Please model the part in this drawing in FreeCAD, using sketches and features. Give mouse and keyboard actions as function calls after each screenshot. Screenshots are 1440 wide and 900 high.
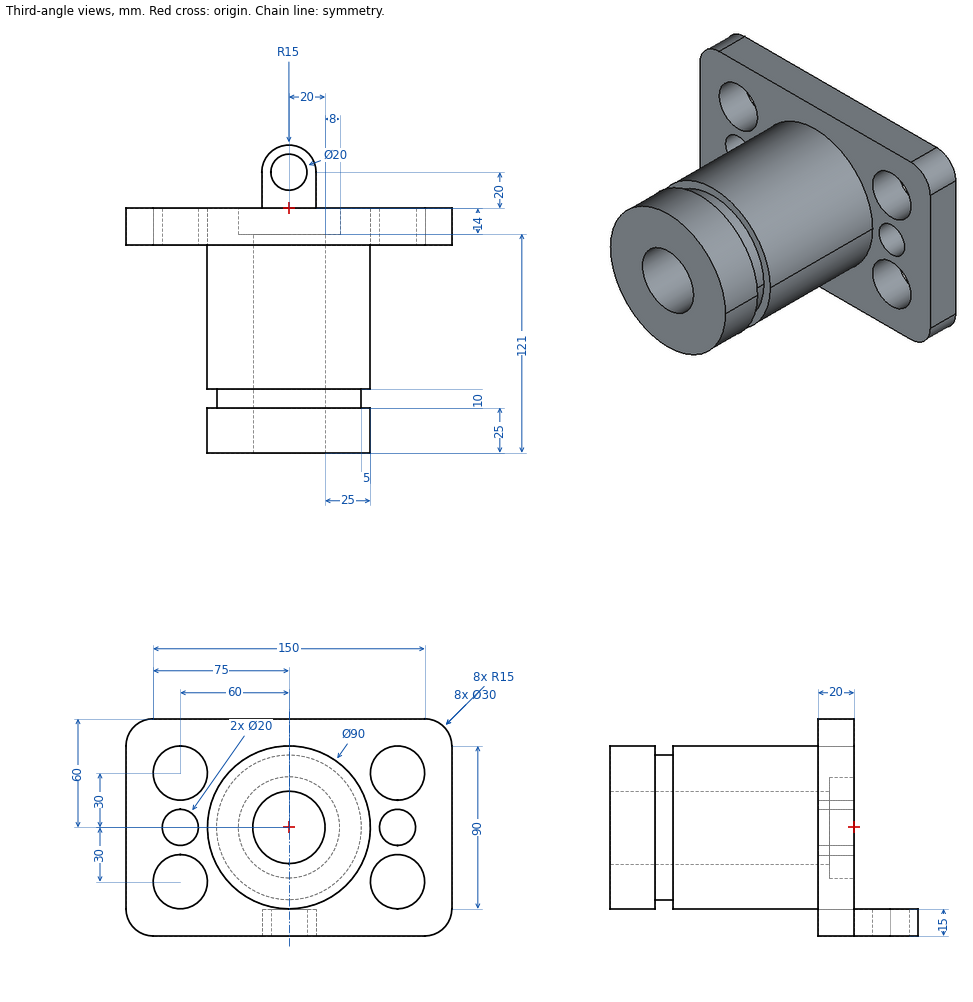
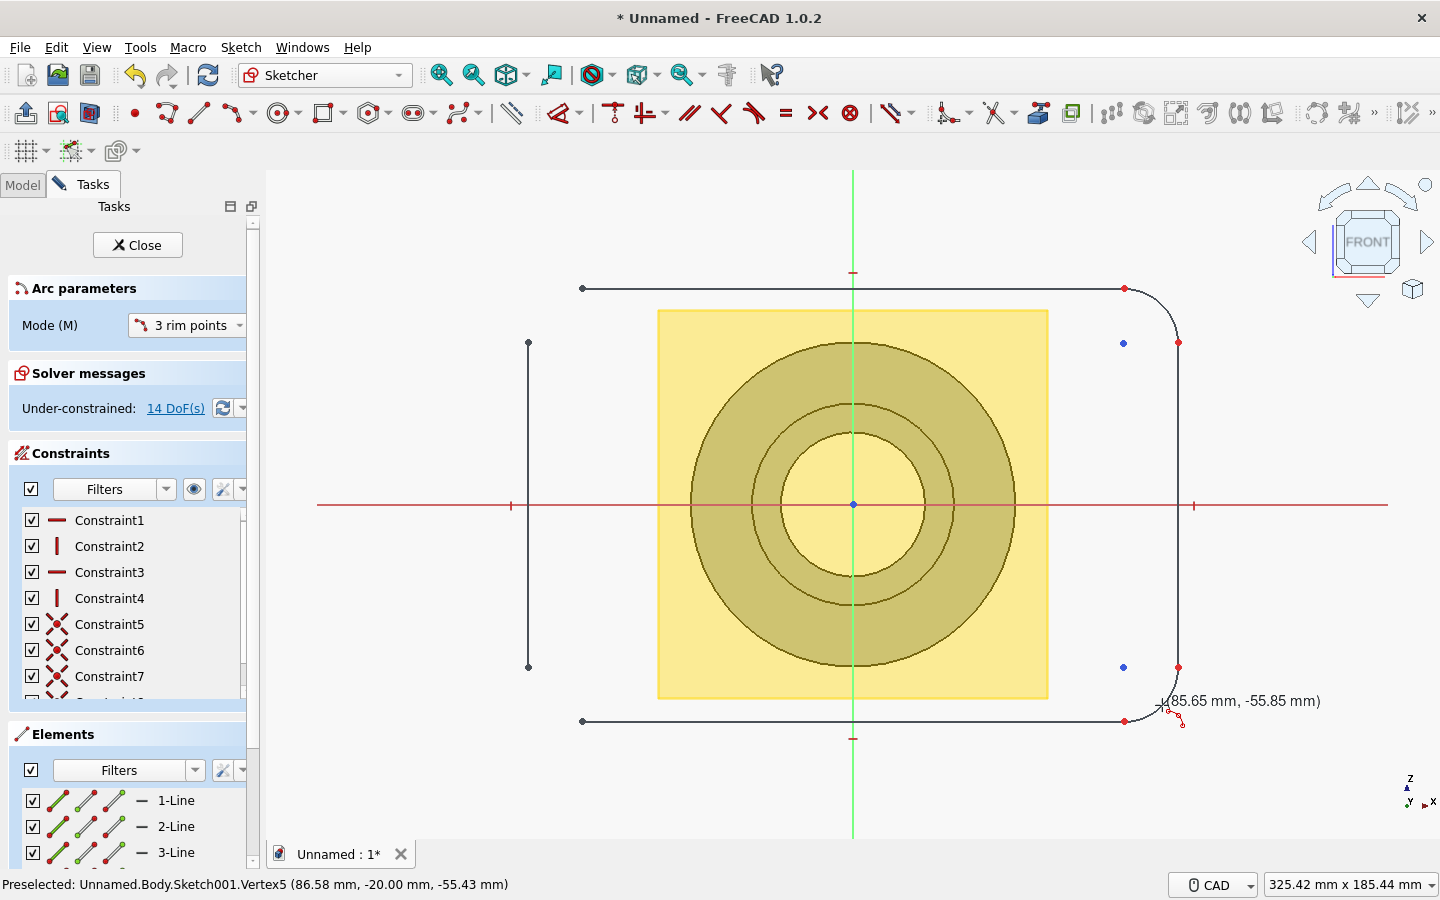
click(582, 722)
click(528, 668)
click(544, 705)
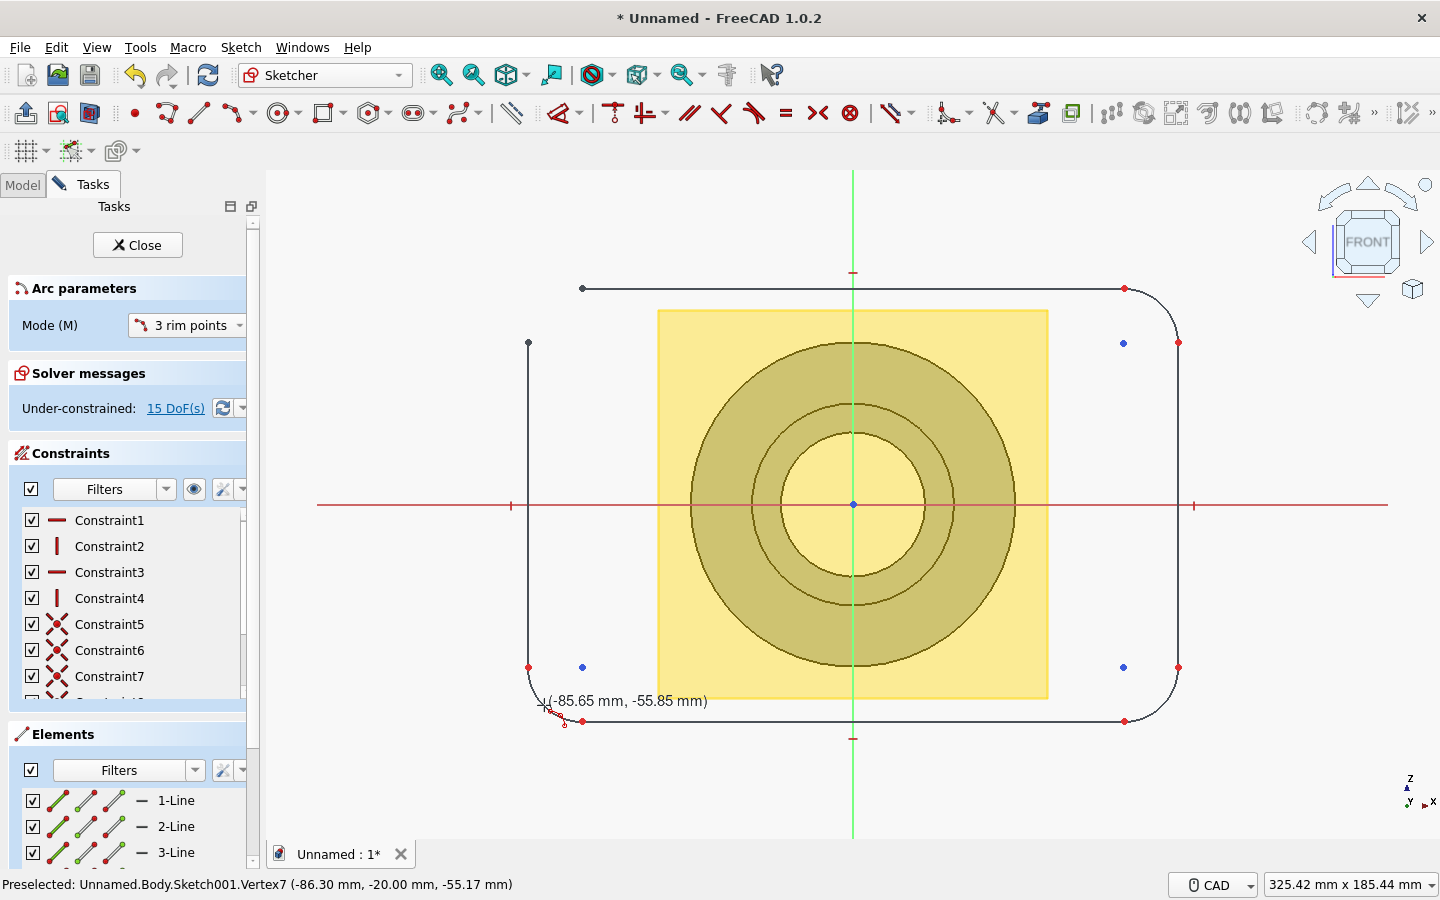
click(528, 343)
click(582, 289)
click(544, 304)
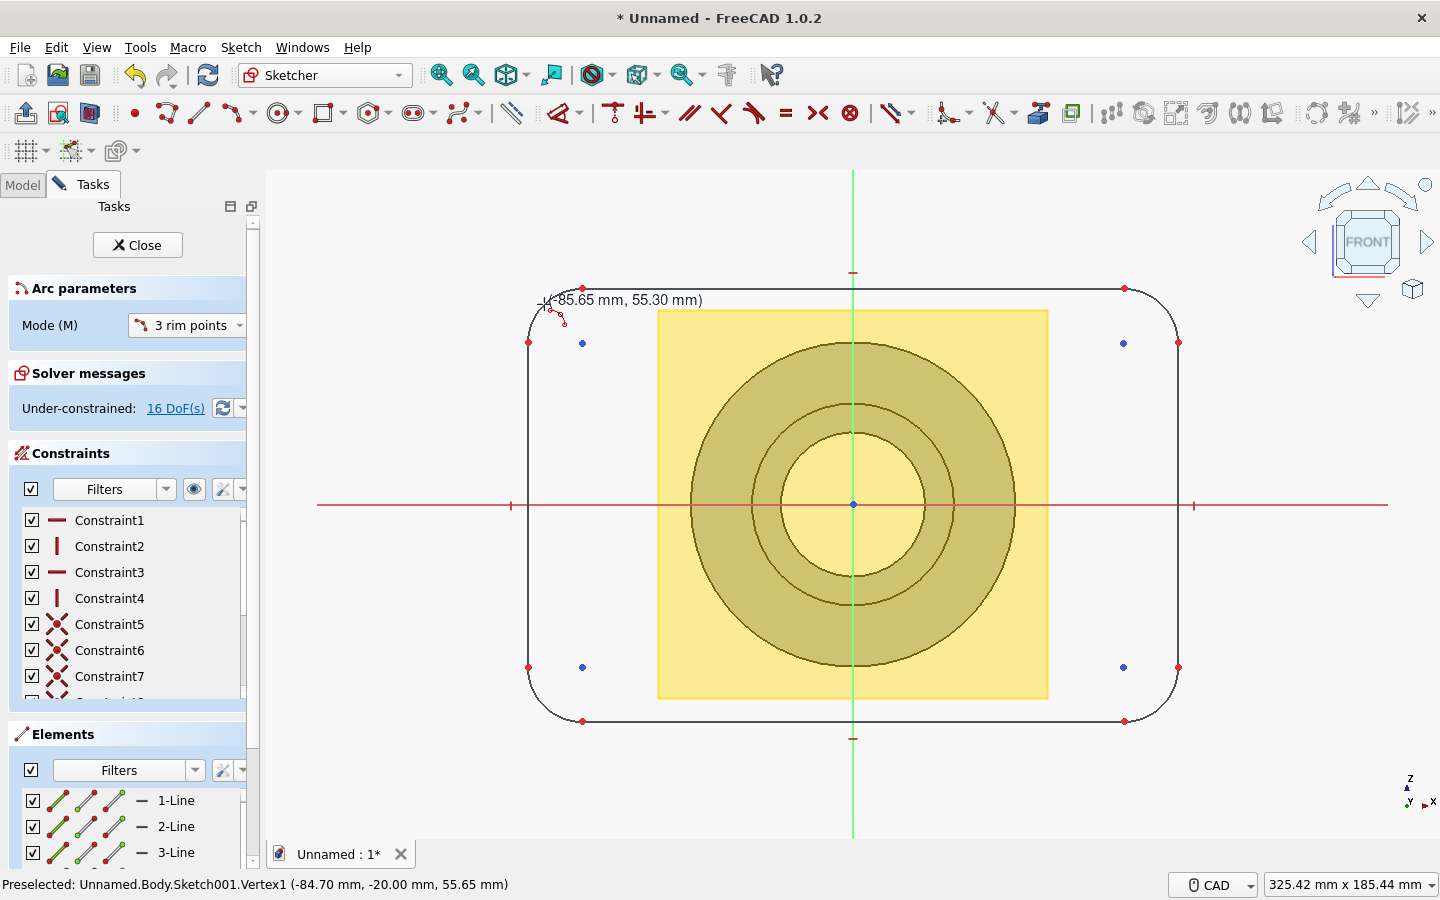
click(278, 114)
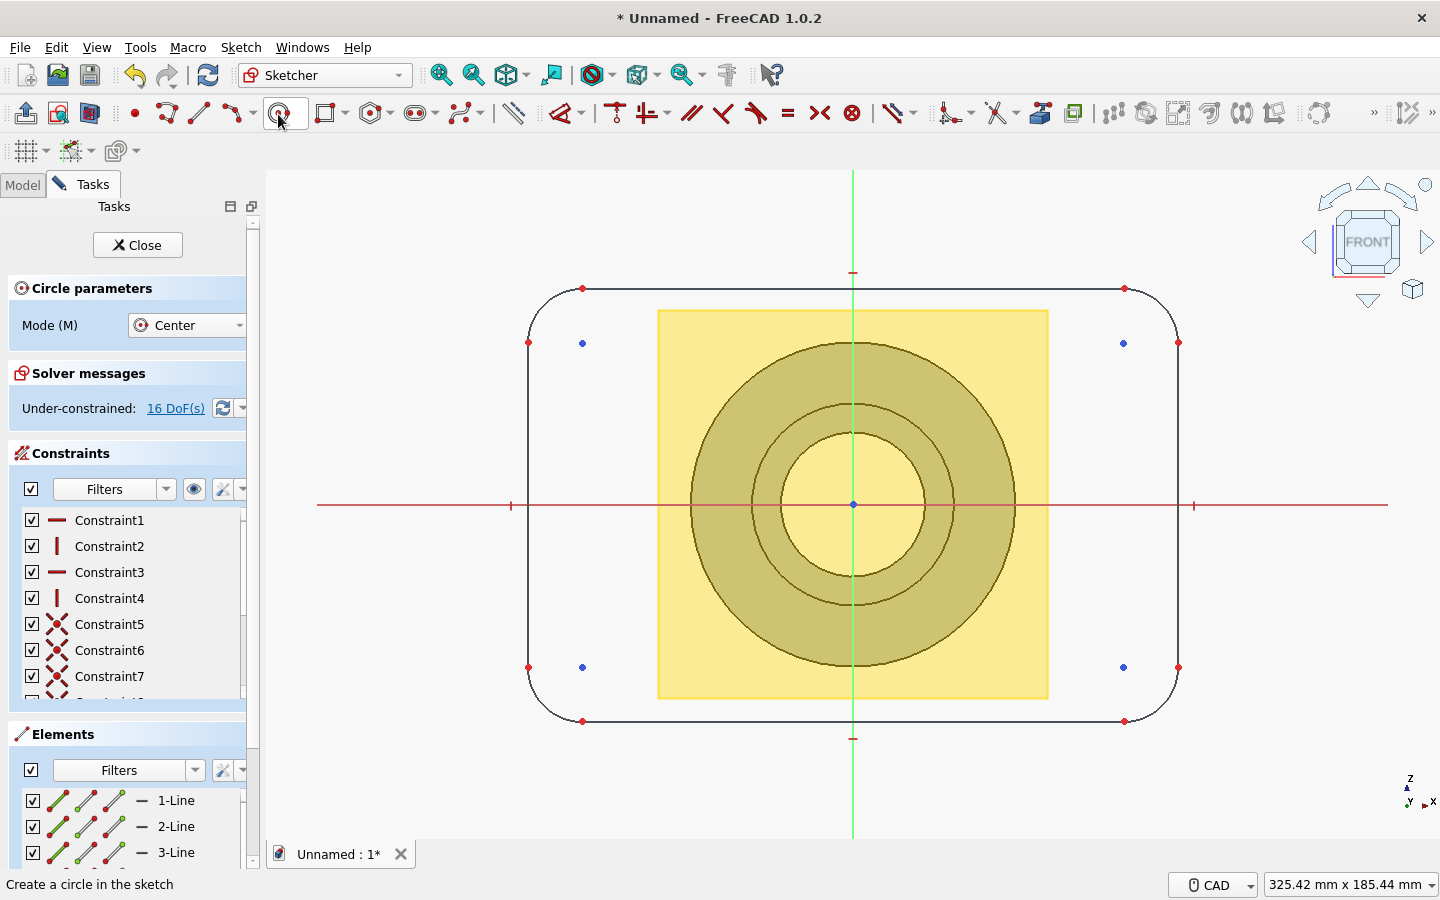
click(637, 396)
move(675, 358)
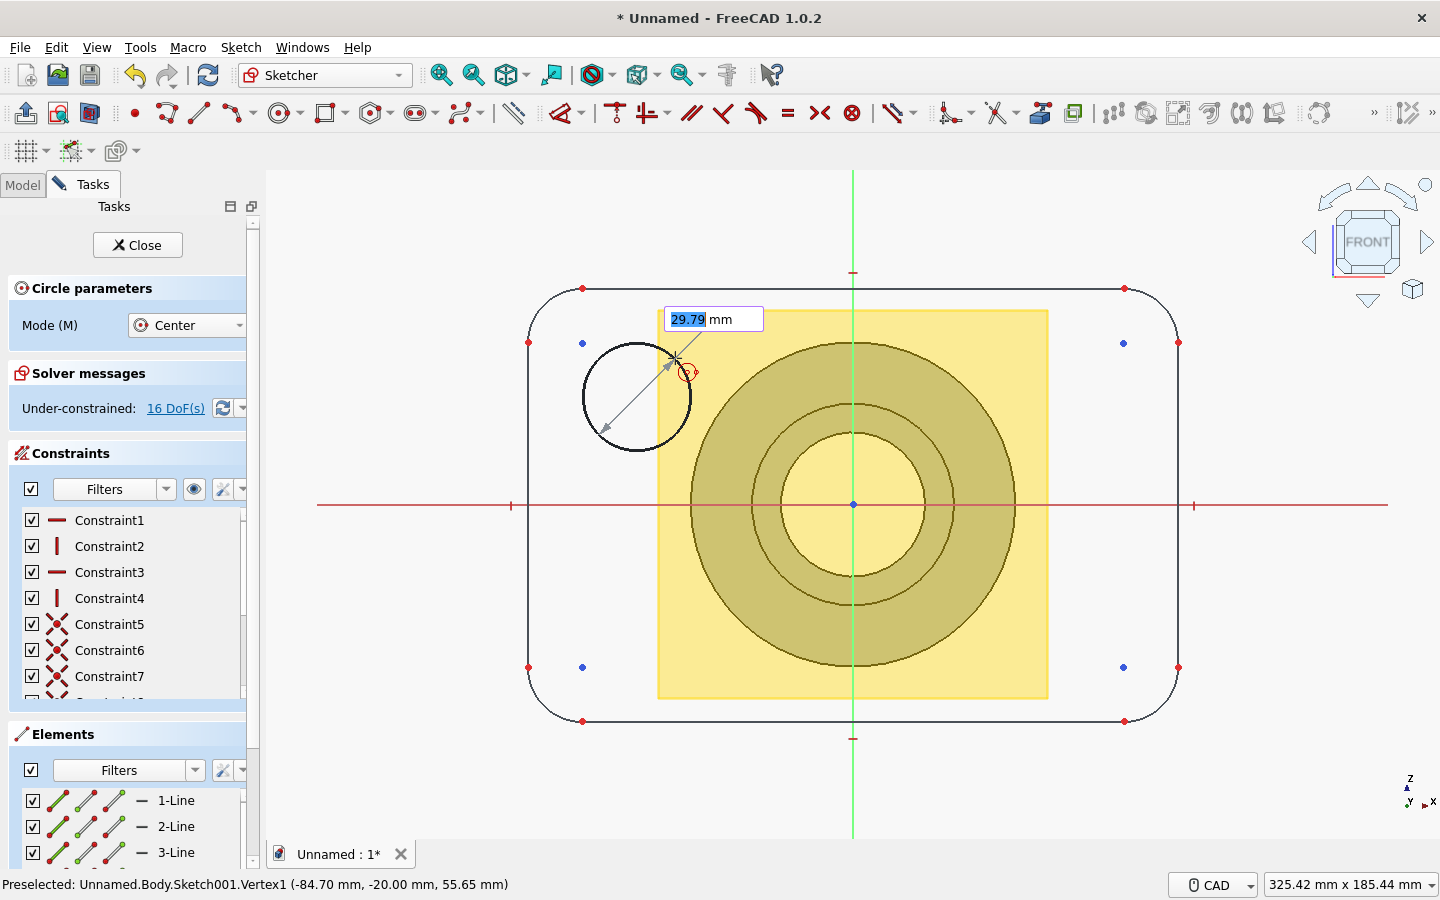
text(30)
key(Return)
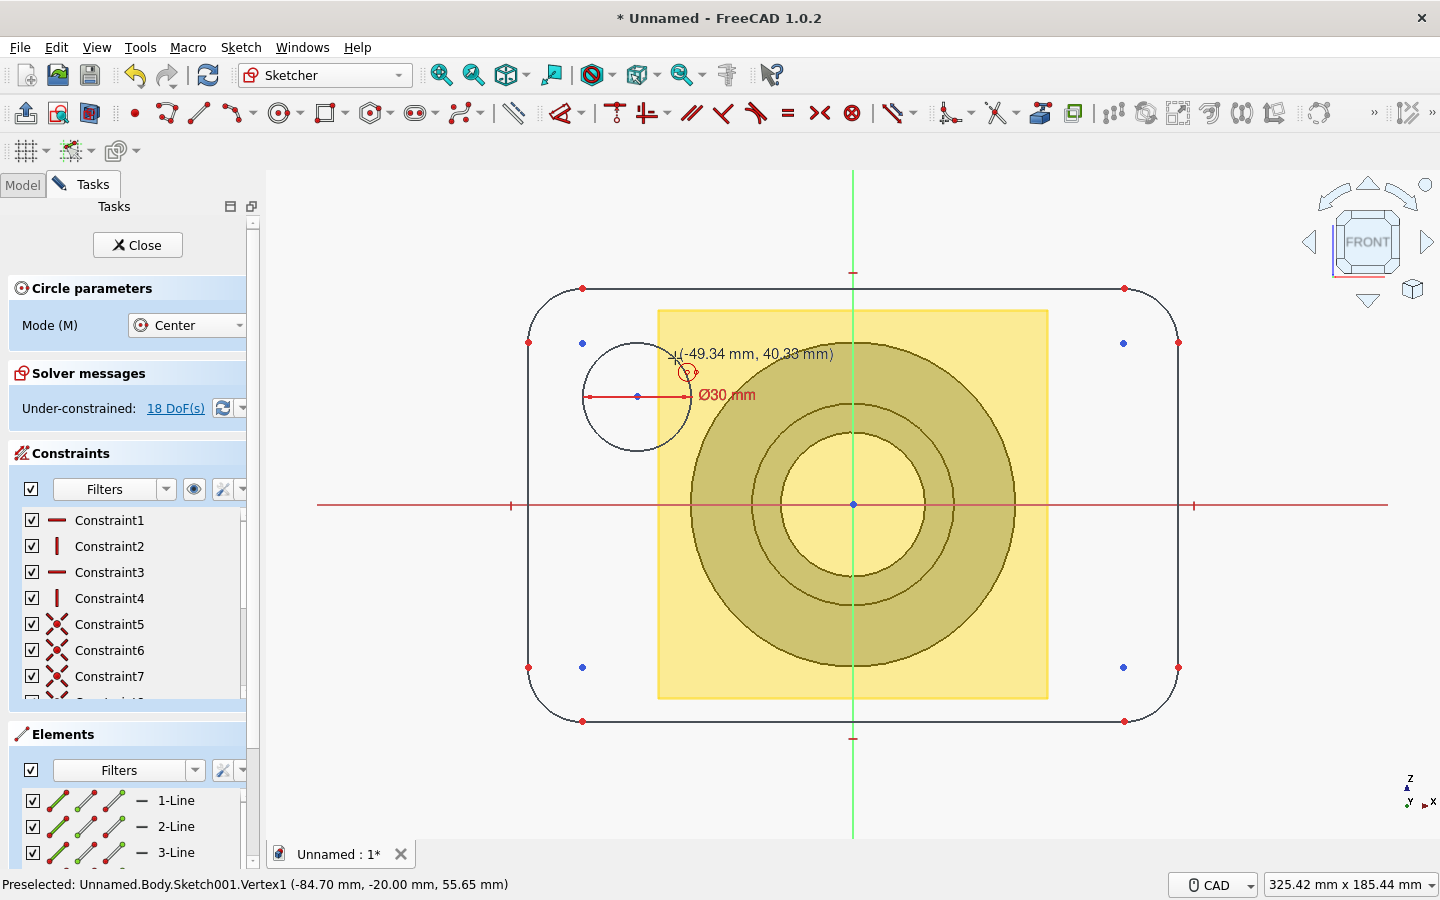
click(1069, 396)
move(1108, 358)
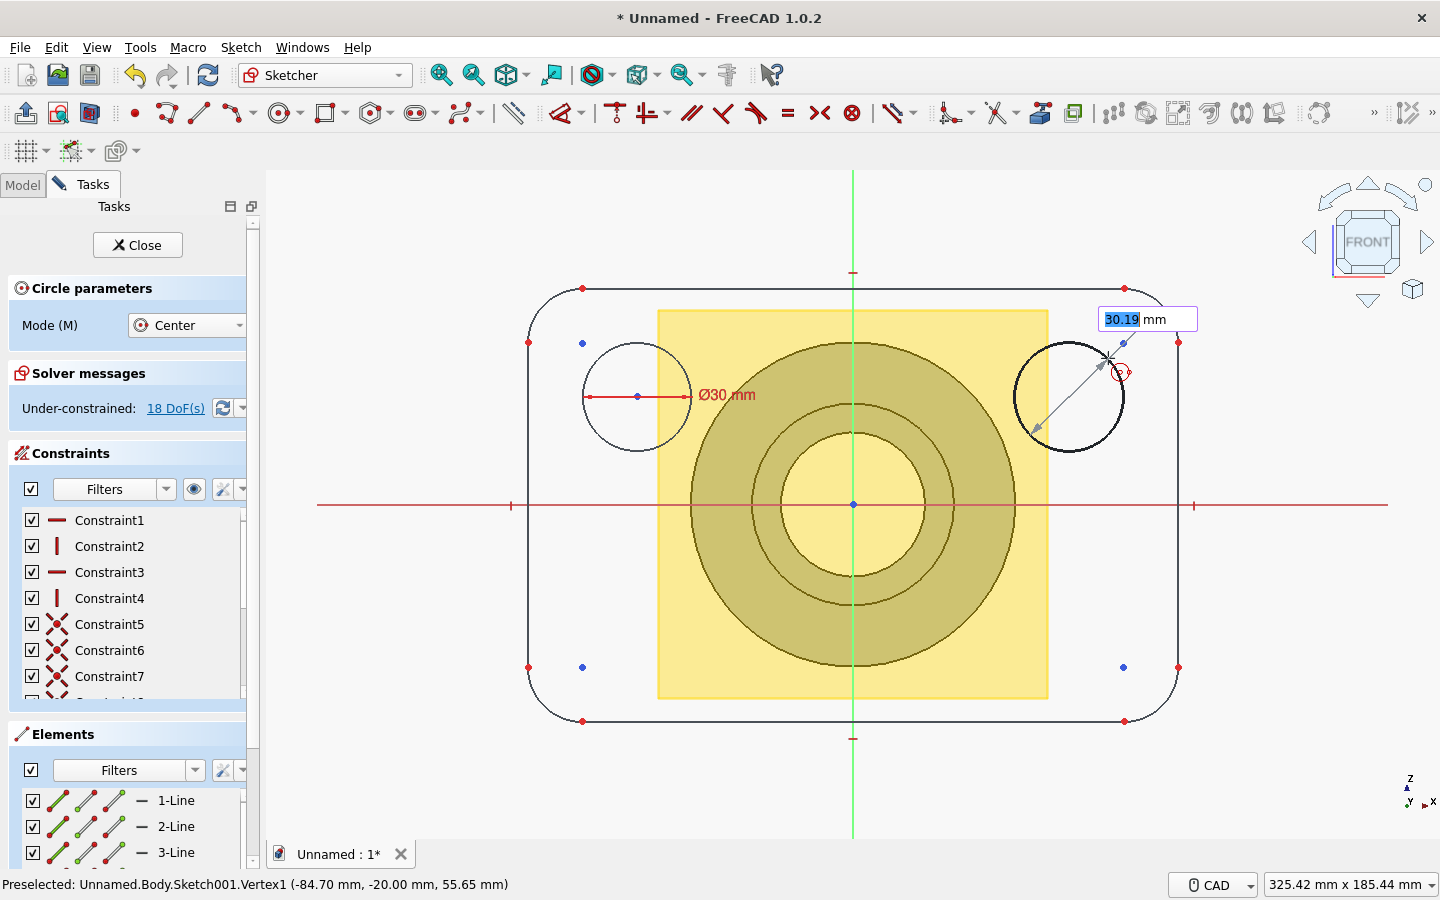
text(30)
key(Return)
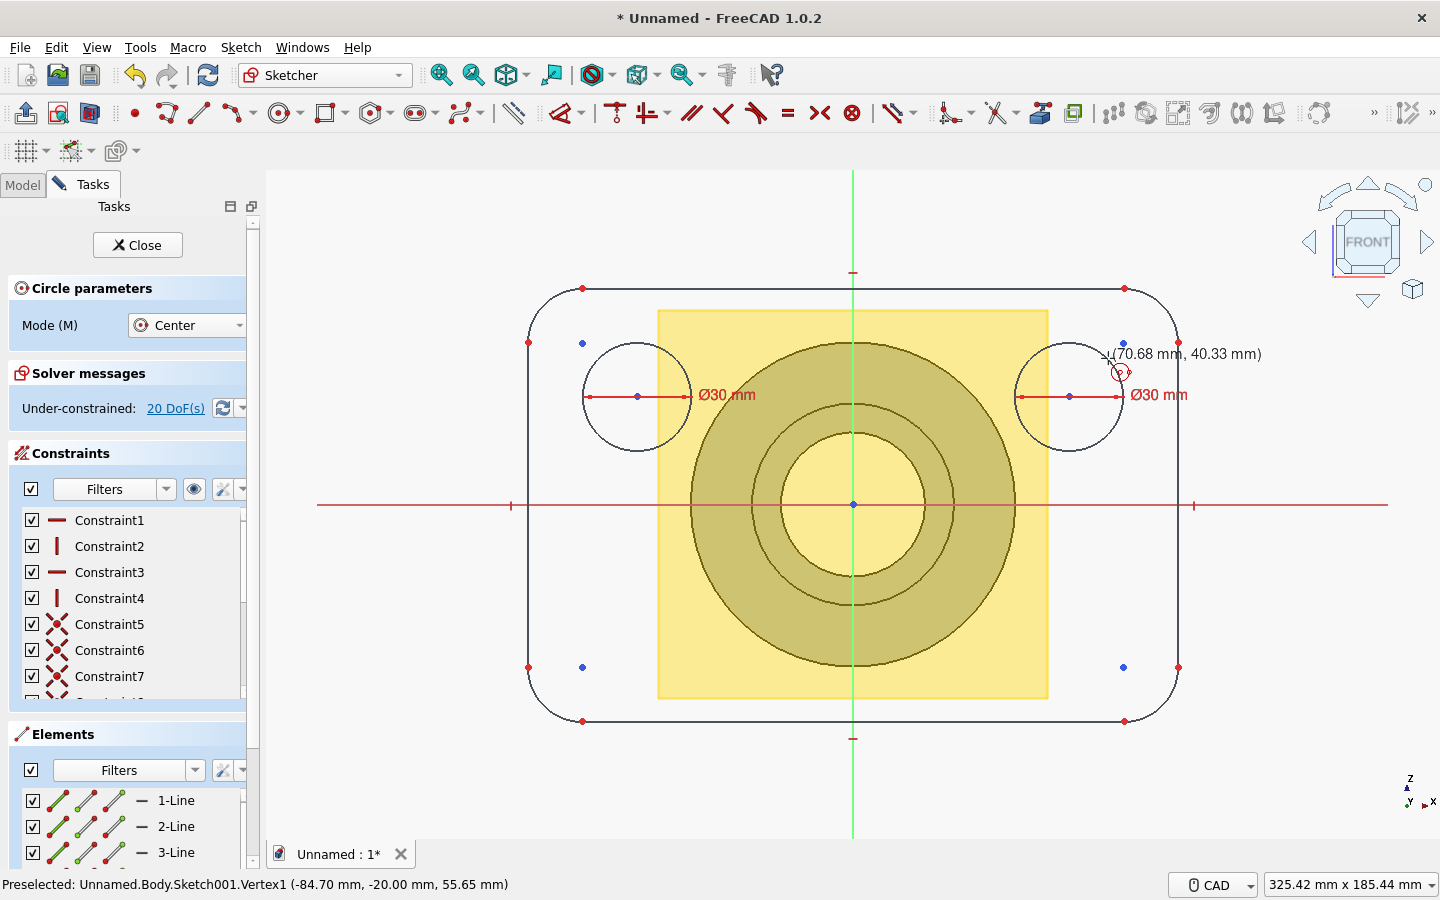
click(637, 504)
move(662, 479)